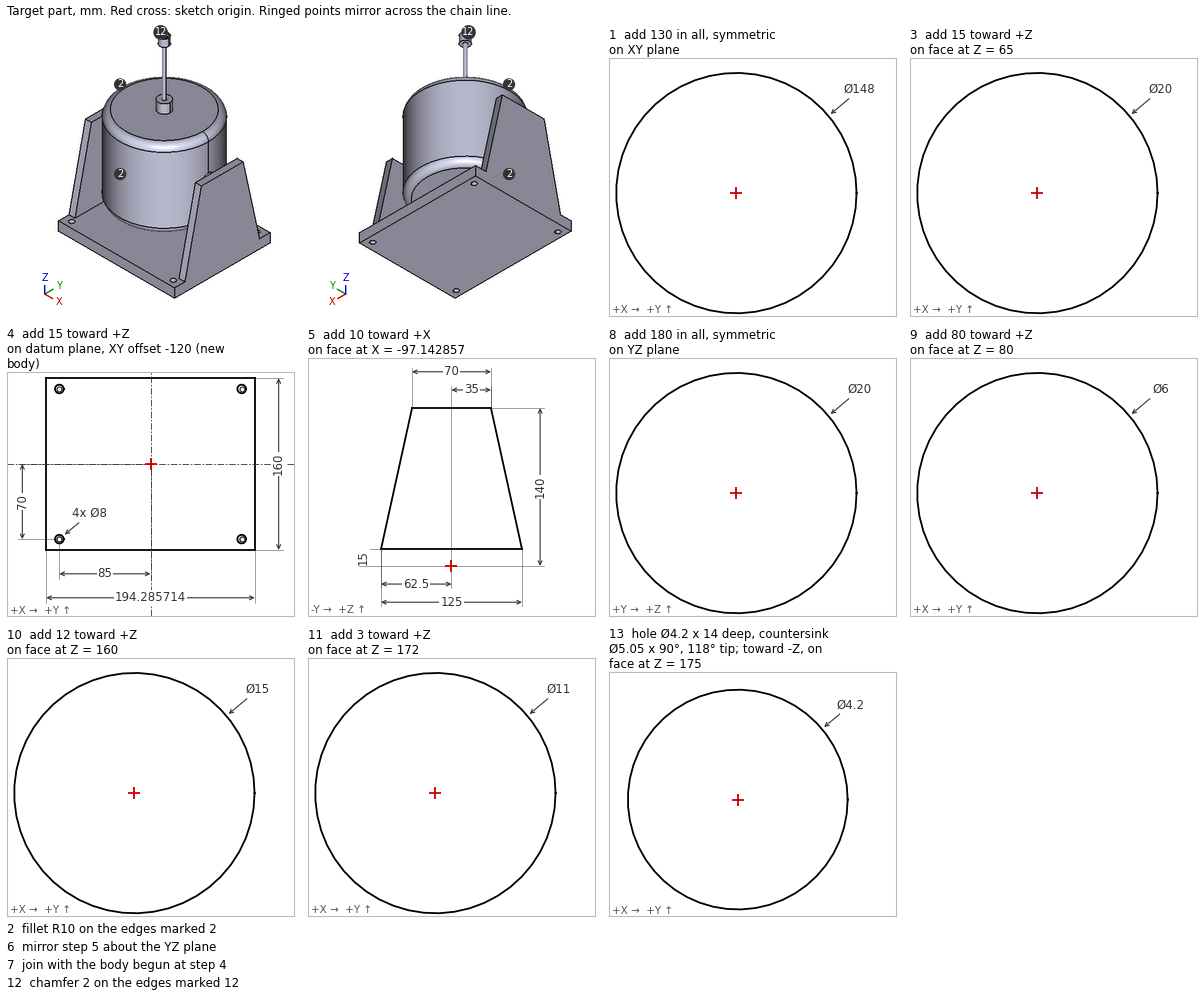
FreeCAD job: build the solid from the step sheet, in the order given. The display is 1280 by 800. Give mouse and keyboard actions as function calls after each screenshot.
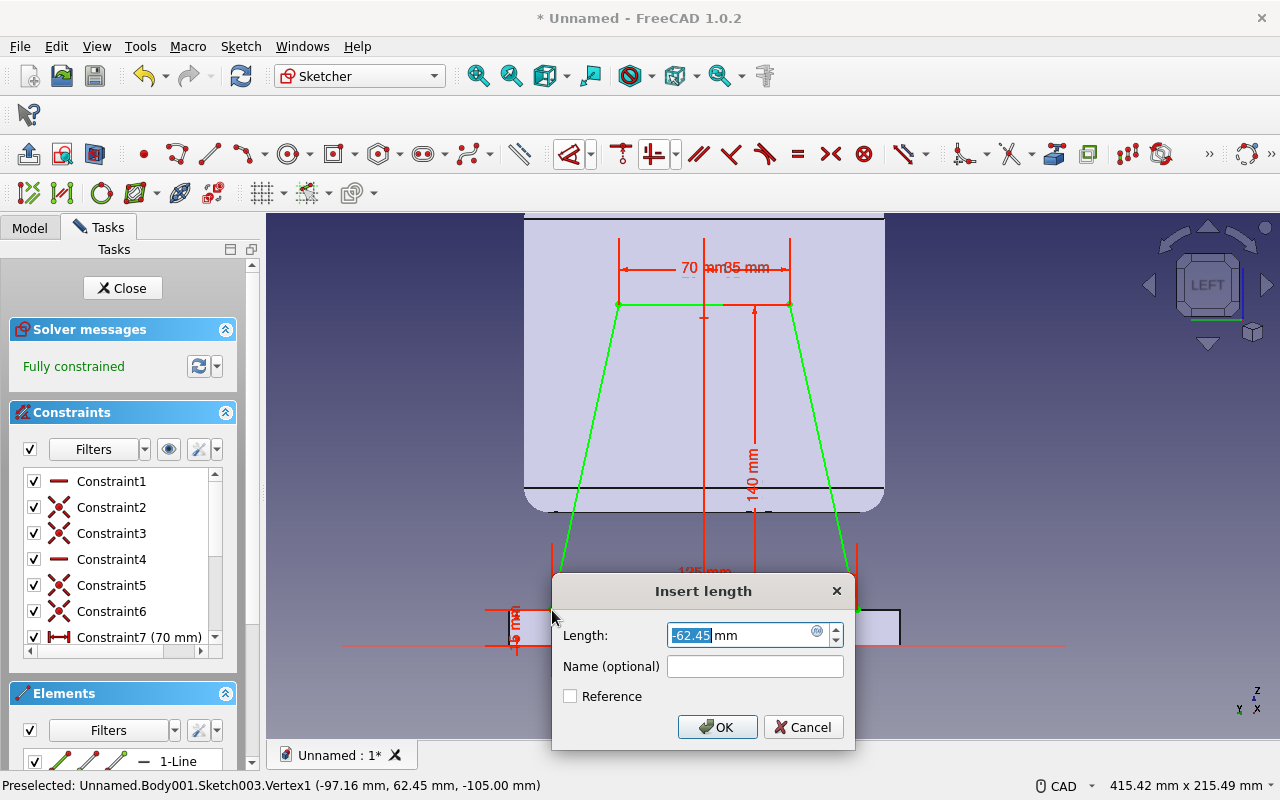
text(-62.5)
key(Return)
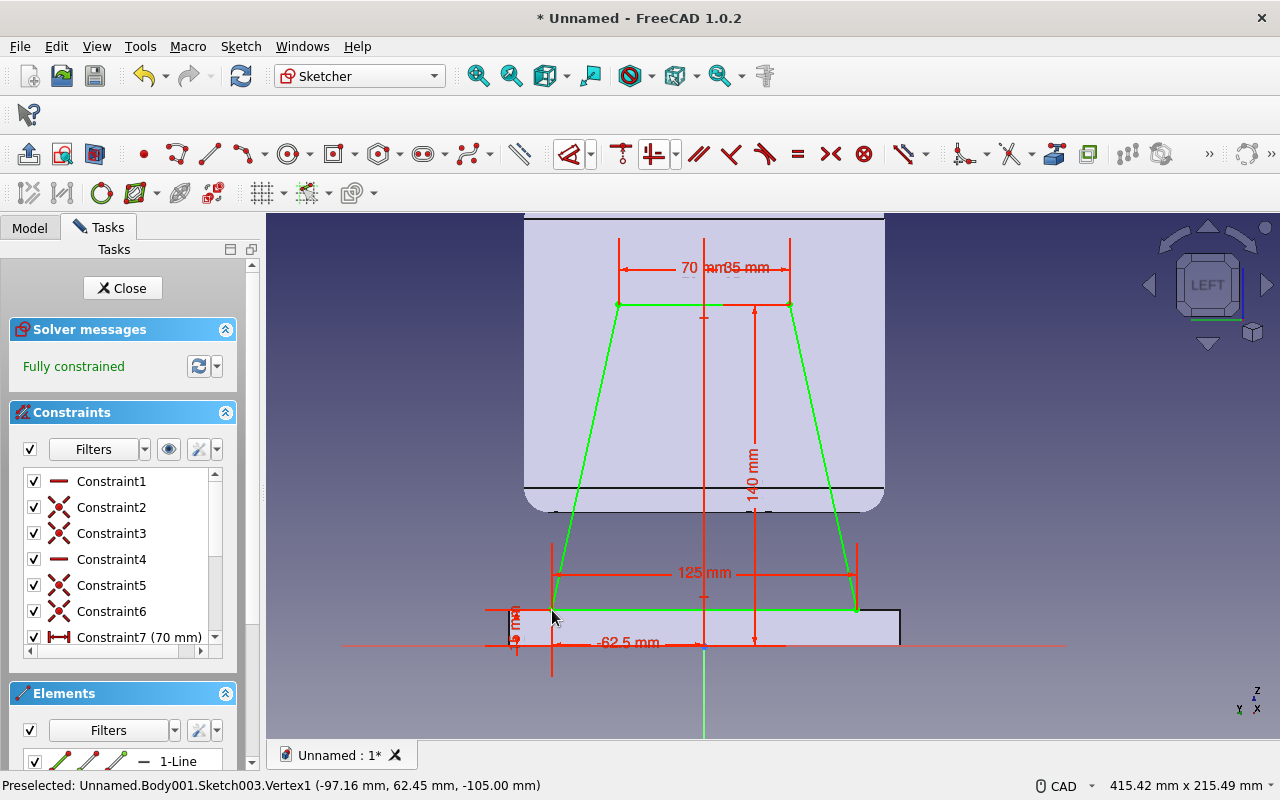
click(123, 288)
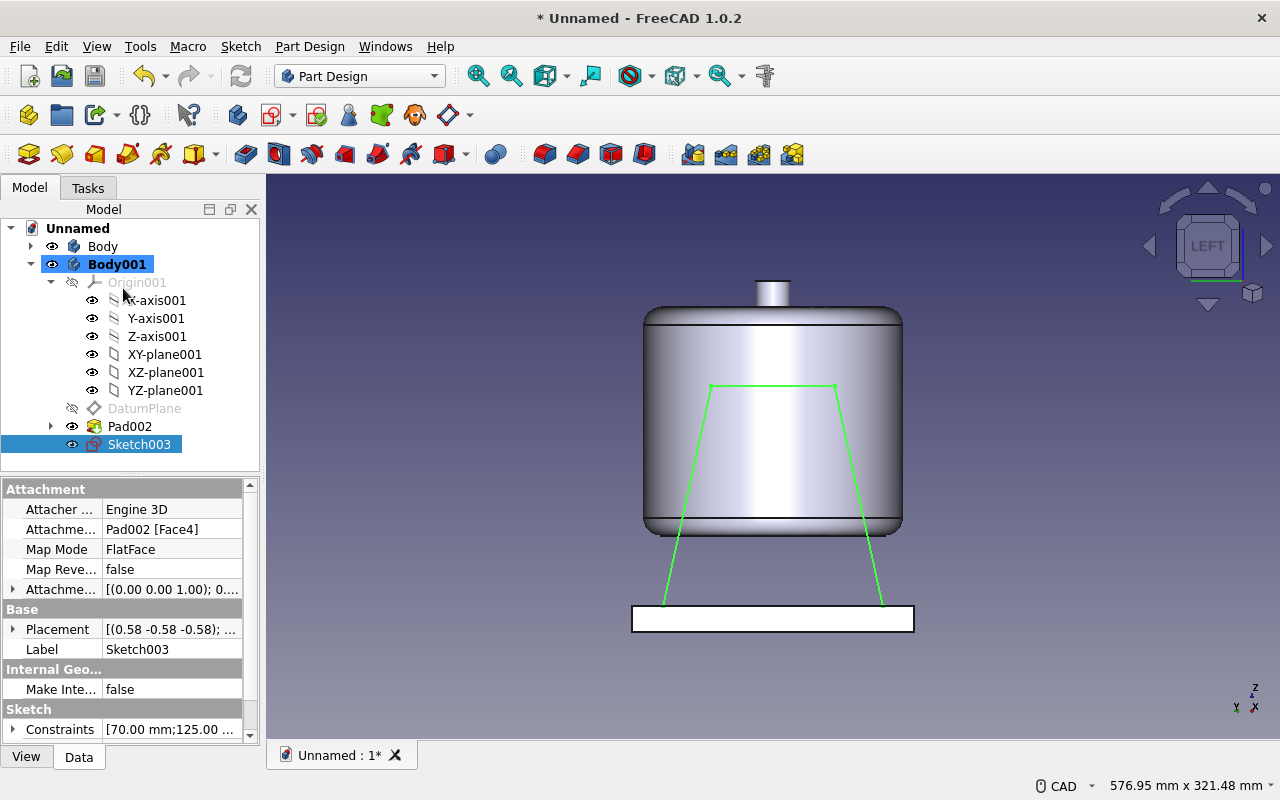
click(29, 154)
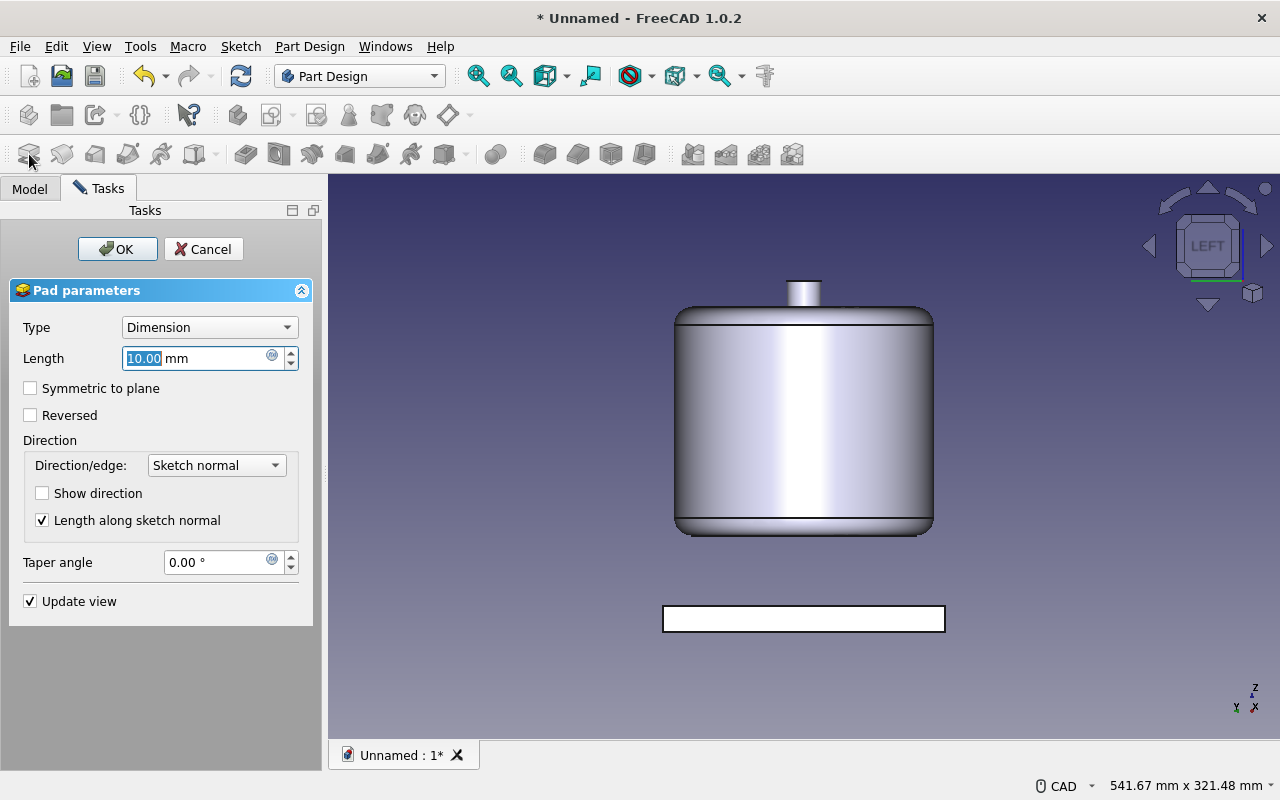
text(10)
key(Tab)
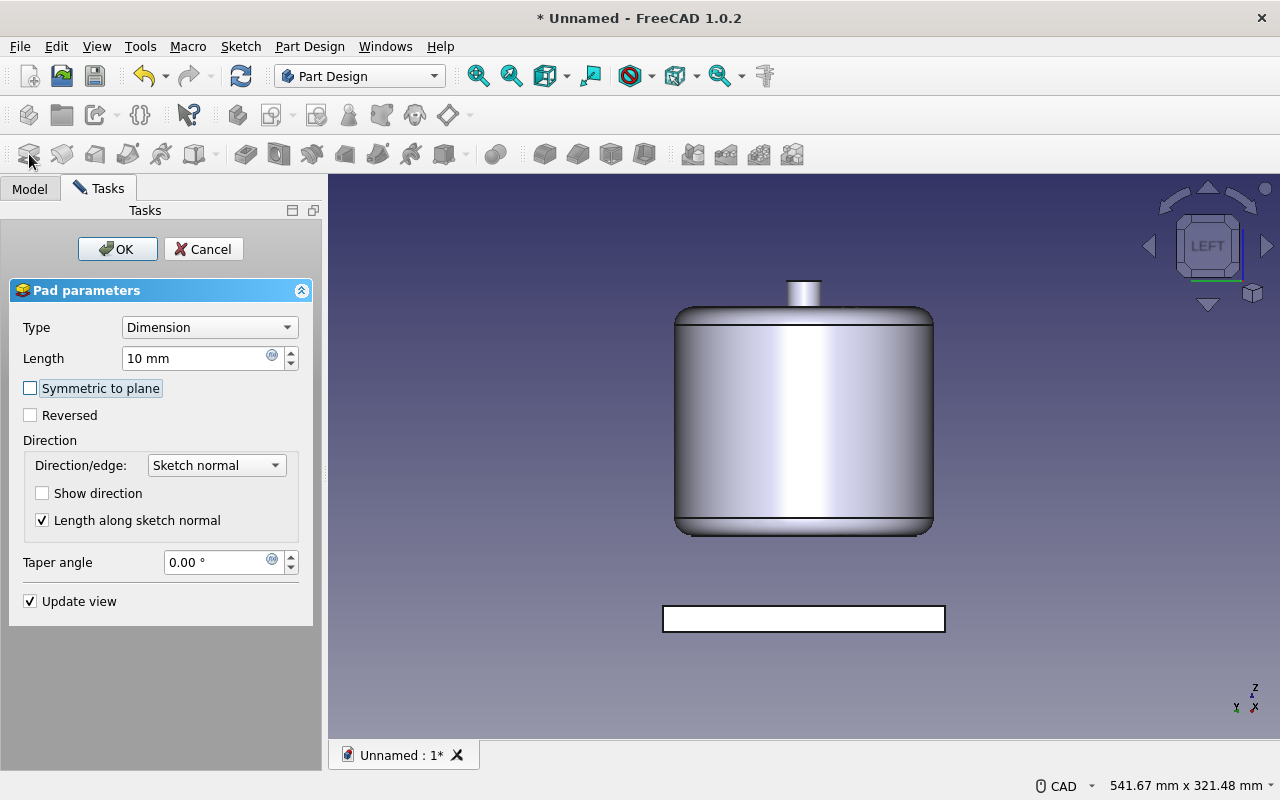
click(31, 415)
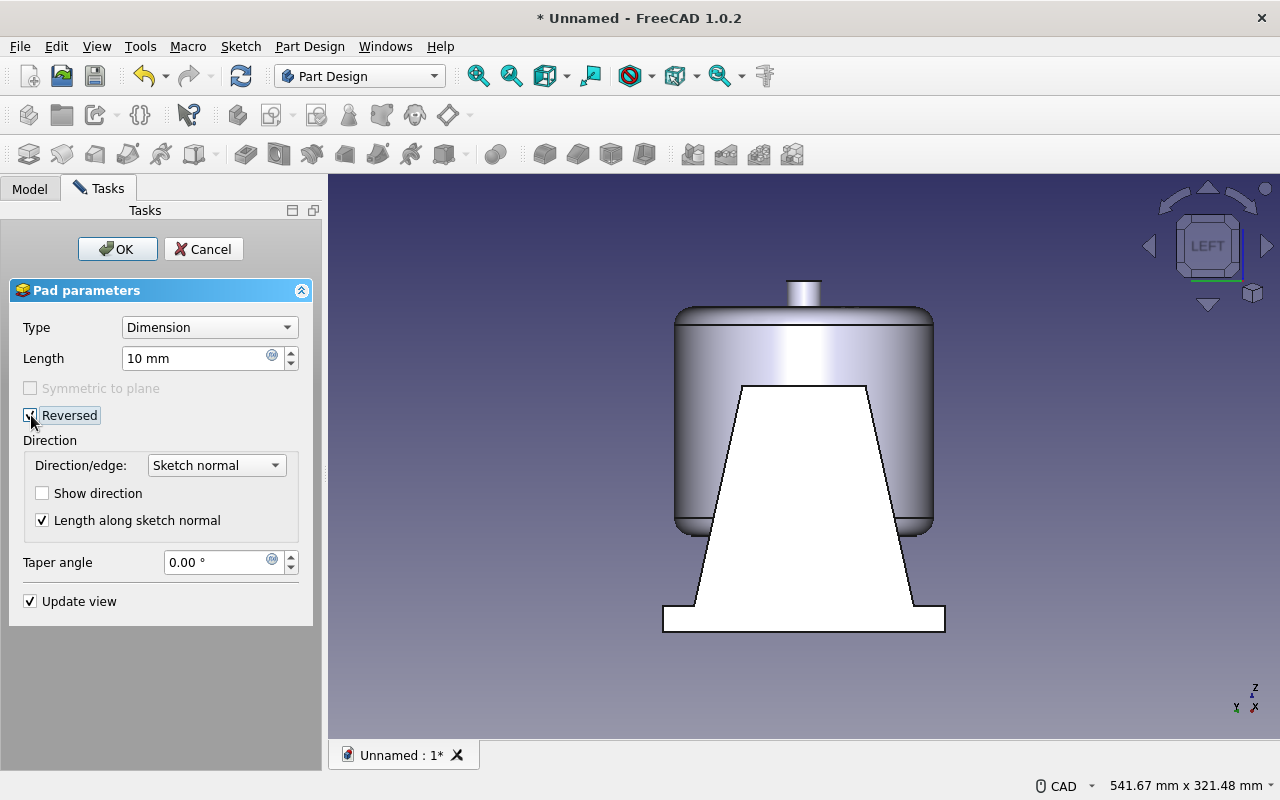
click(118, 249)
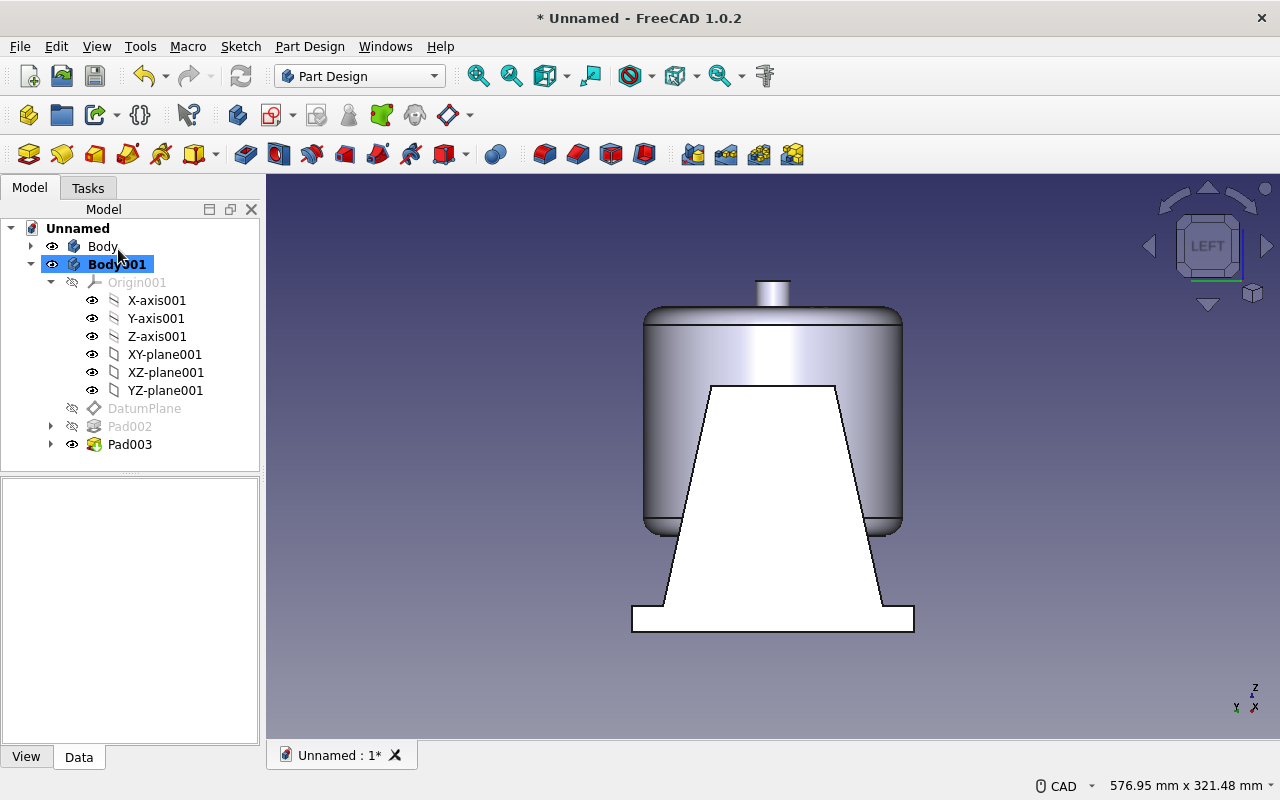
click(479, 76)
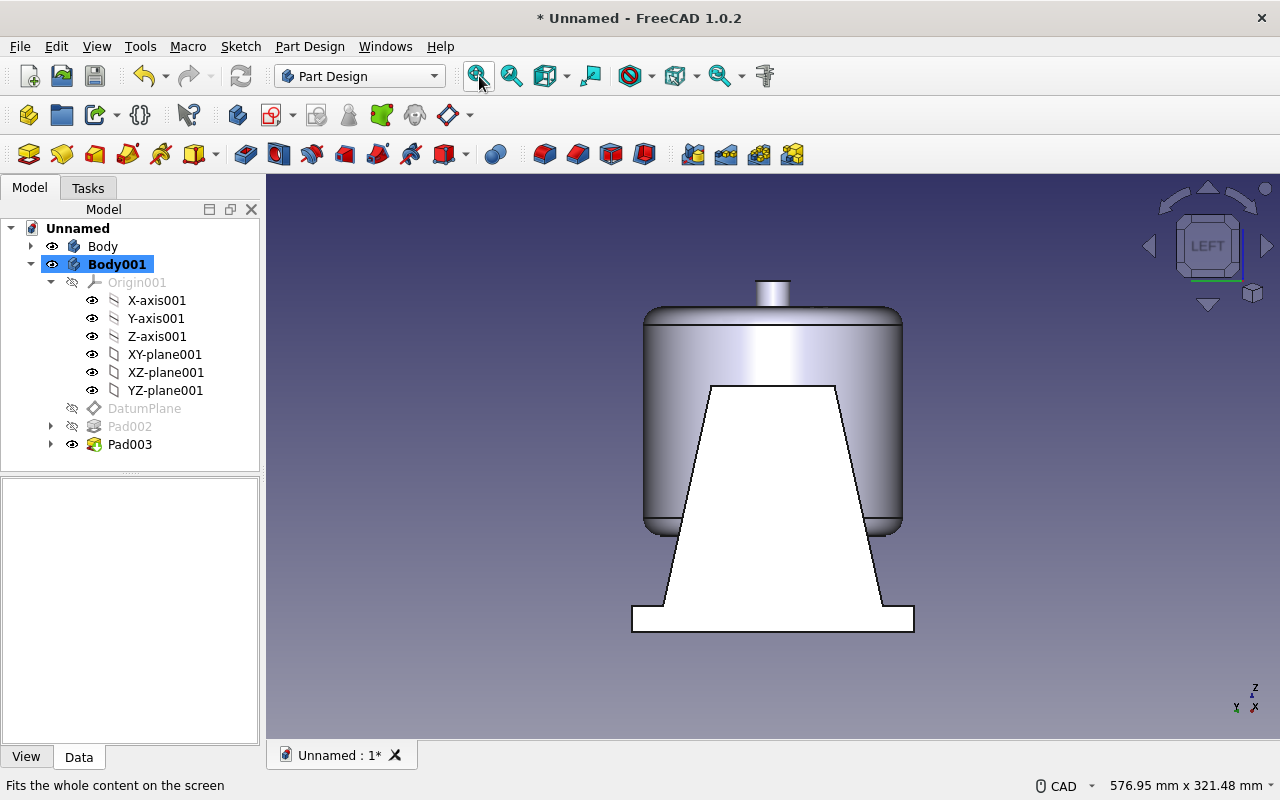
click(117, 444)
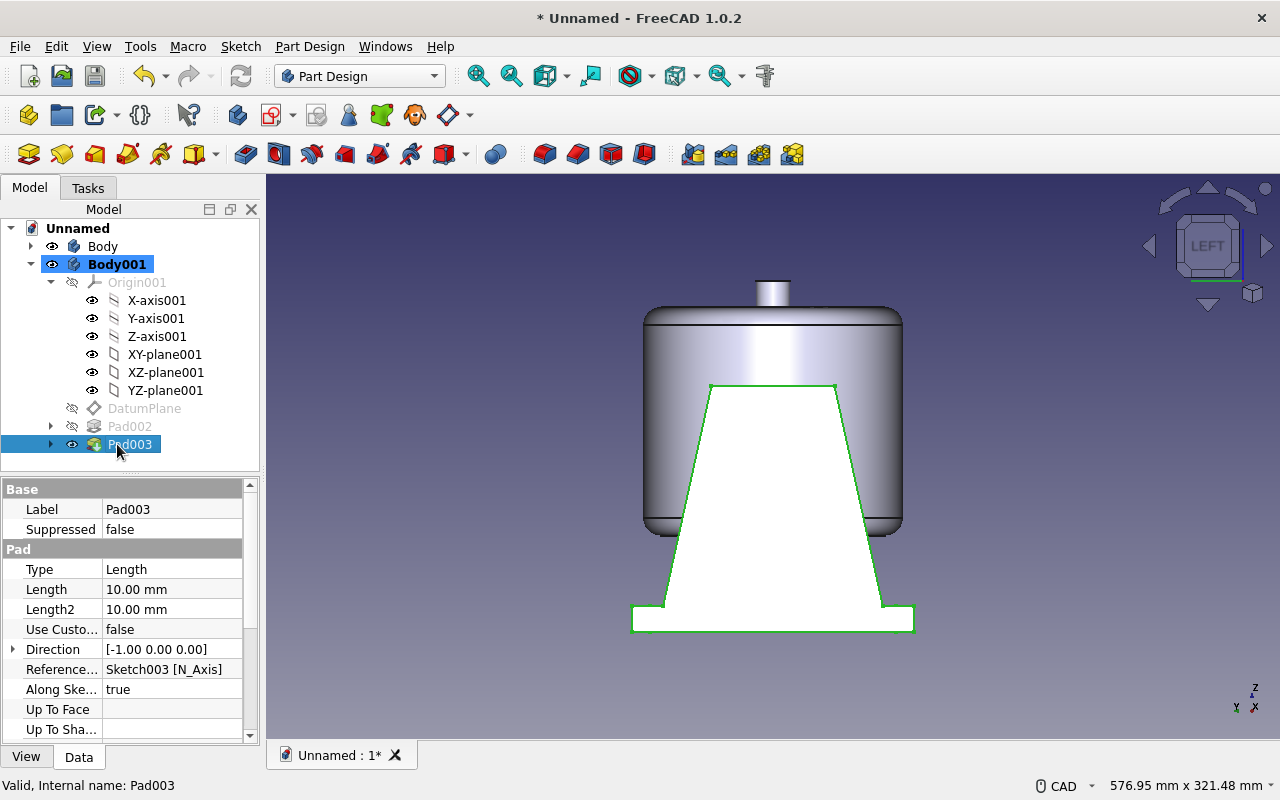
click(693, 154)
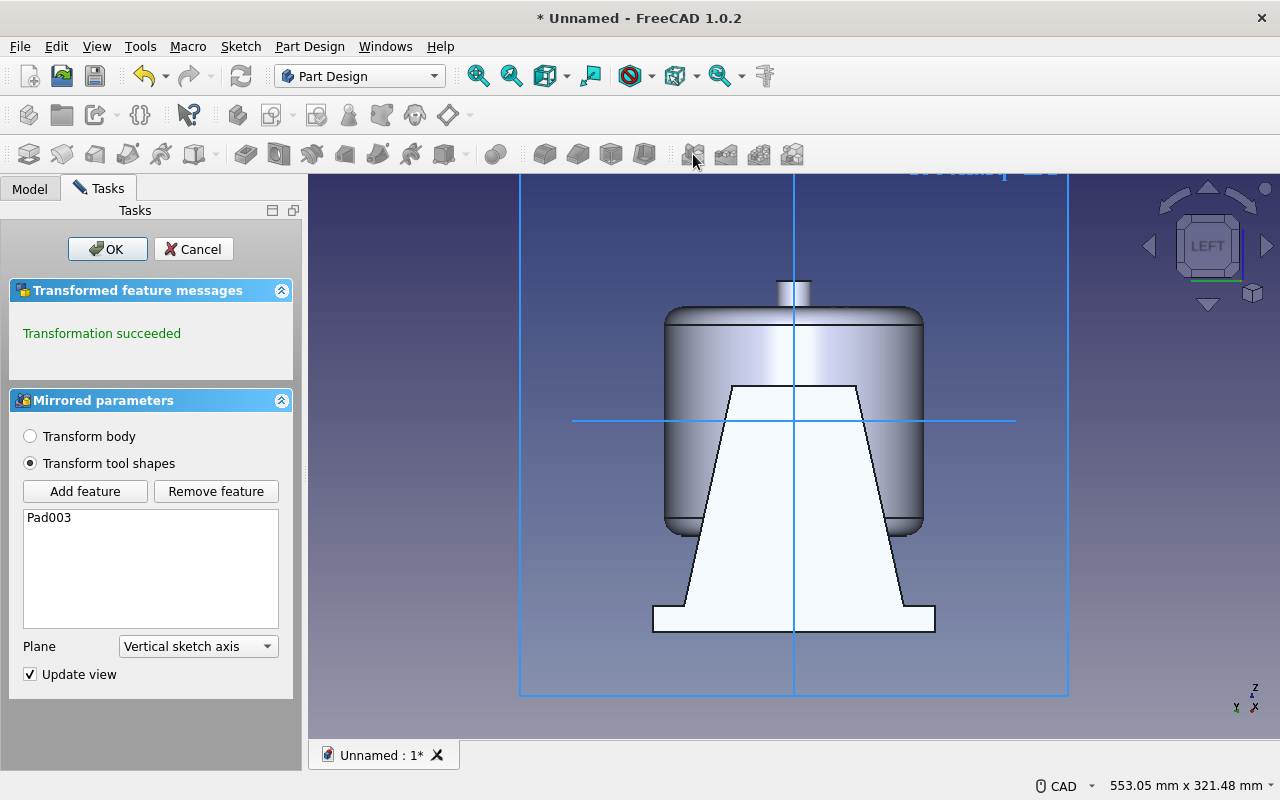
click(199, 646)